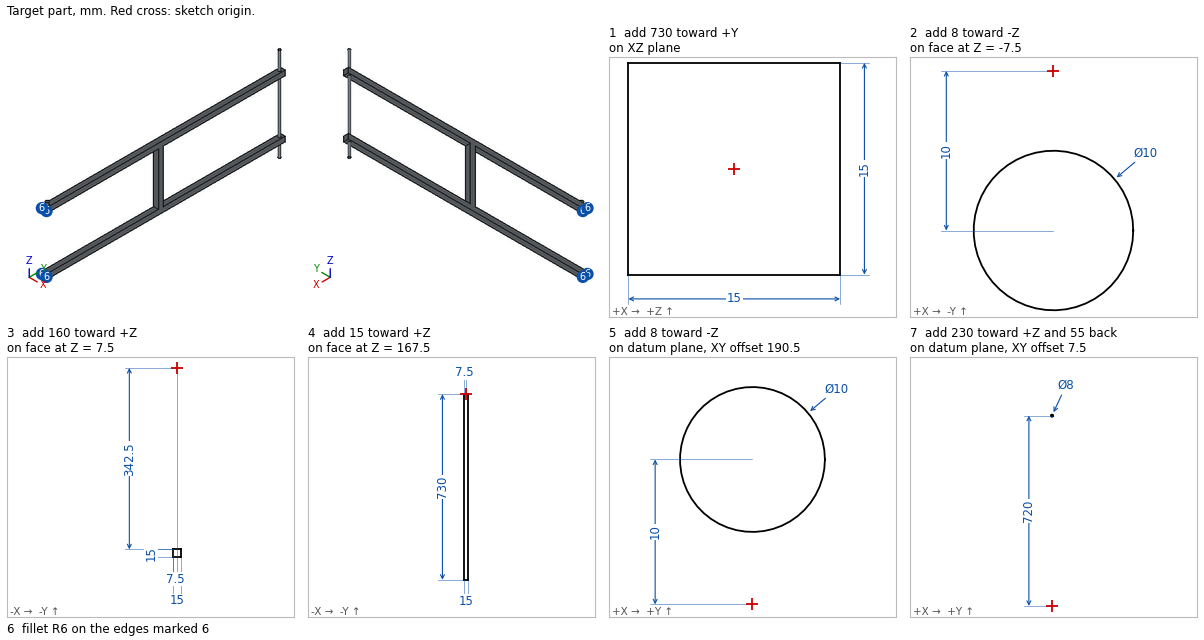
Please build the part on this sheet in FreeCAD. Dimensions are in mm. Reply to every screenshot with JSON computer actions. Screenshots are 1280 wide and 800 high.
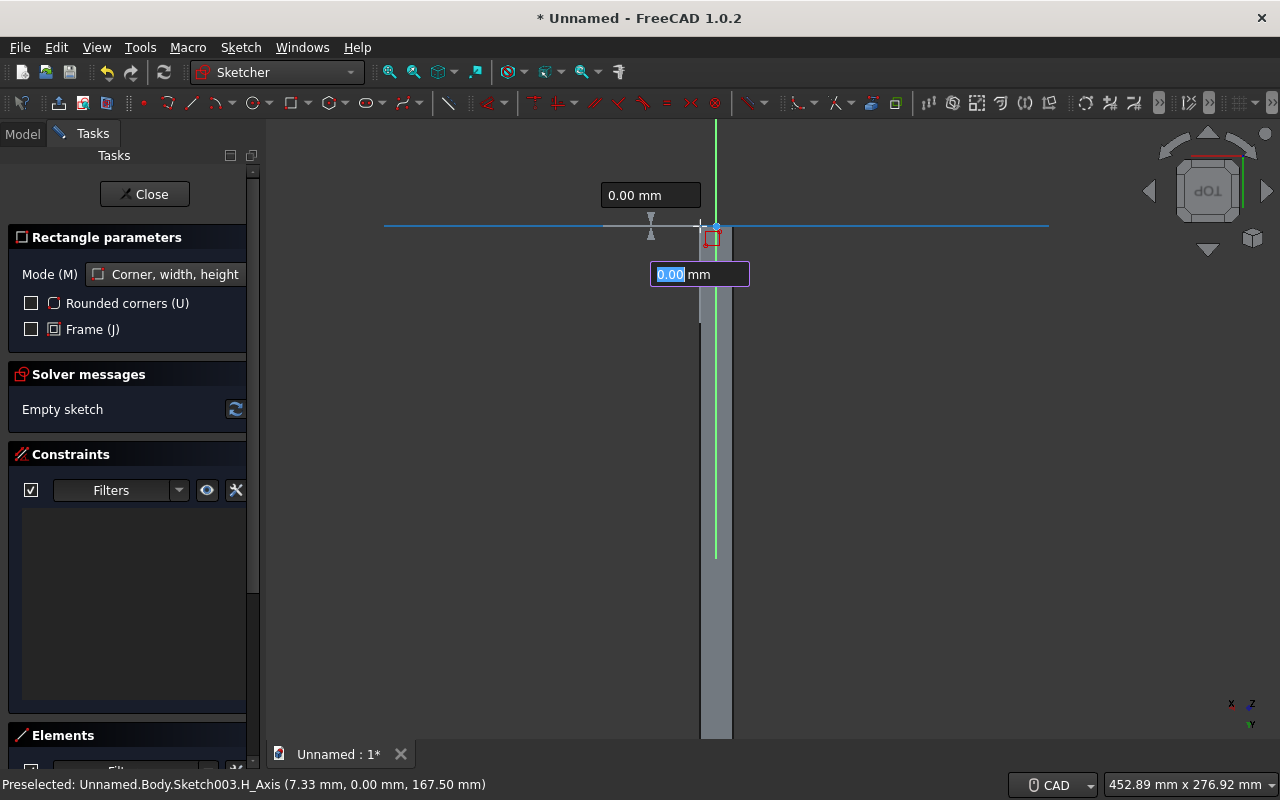
{"action": "scroll", "coordinate": [701, 228], "scroll_direction": "down", "scroll_amount": 7}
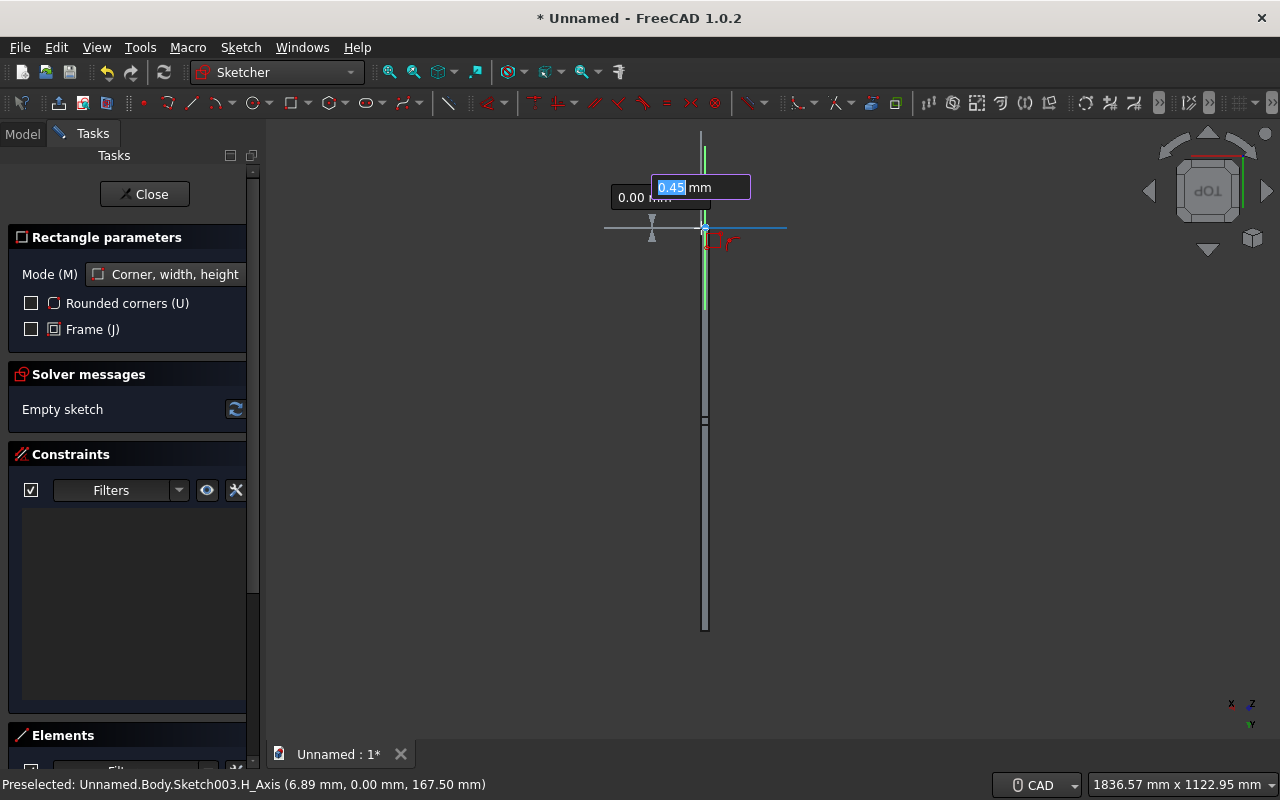
{"action": "scroll", "coordinate": [709, 631], "scroll_direction": "up", "scroll_amount": 7}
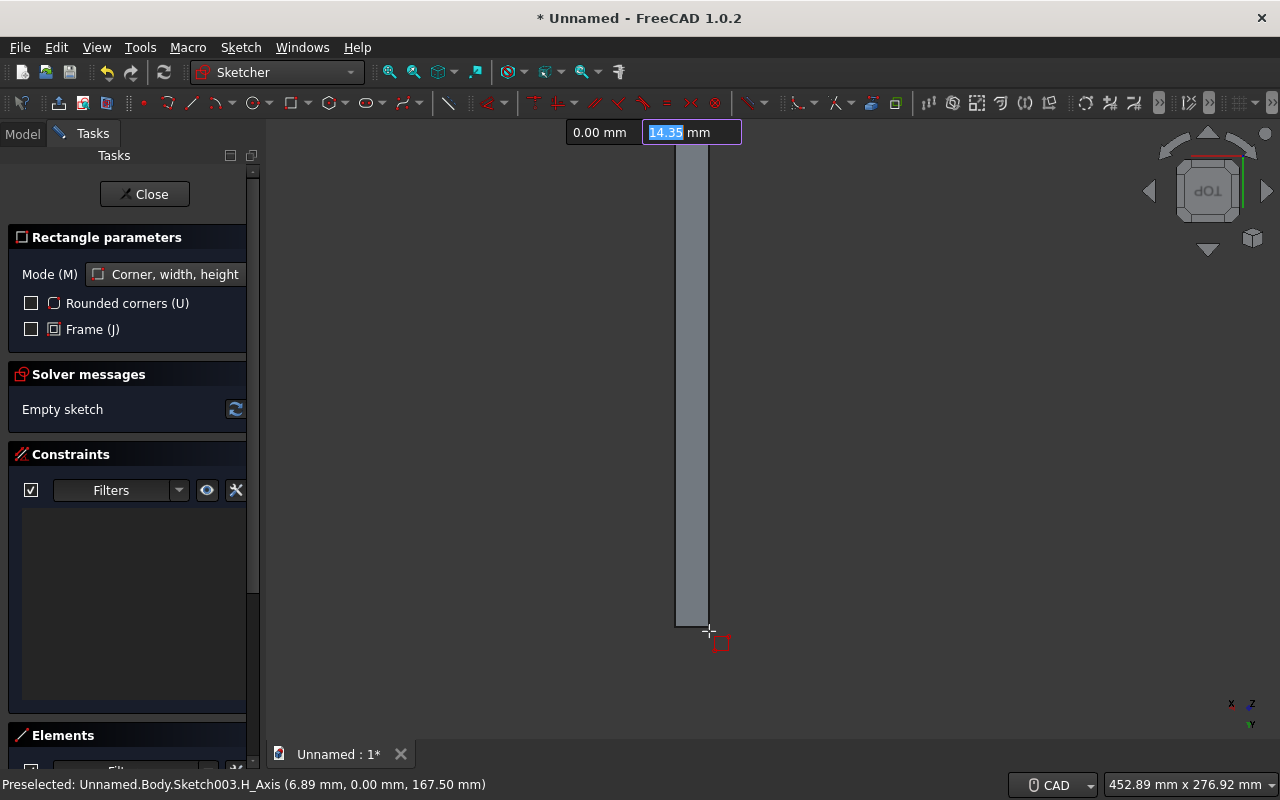
{"action": "left_click", "coordinate": [709, 627]}
{"action": "key", "text": "Escape"}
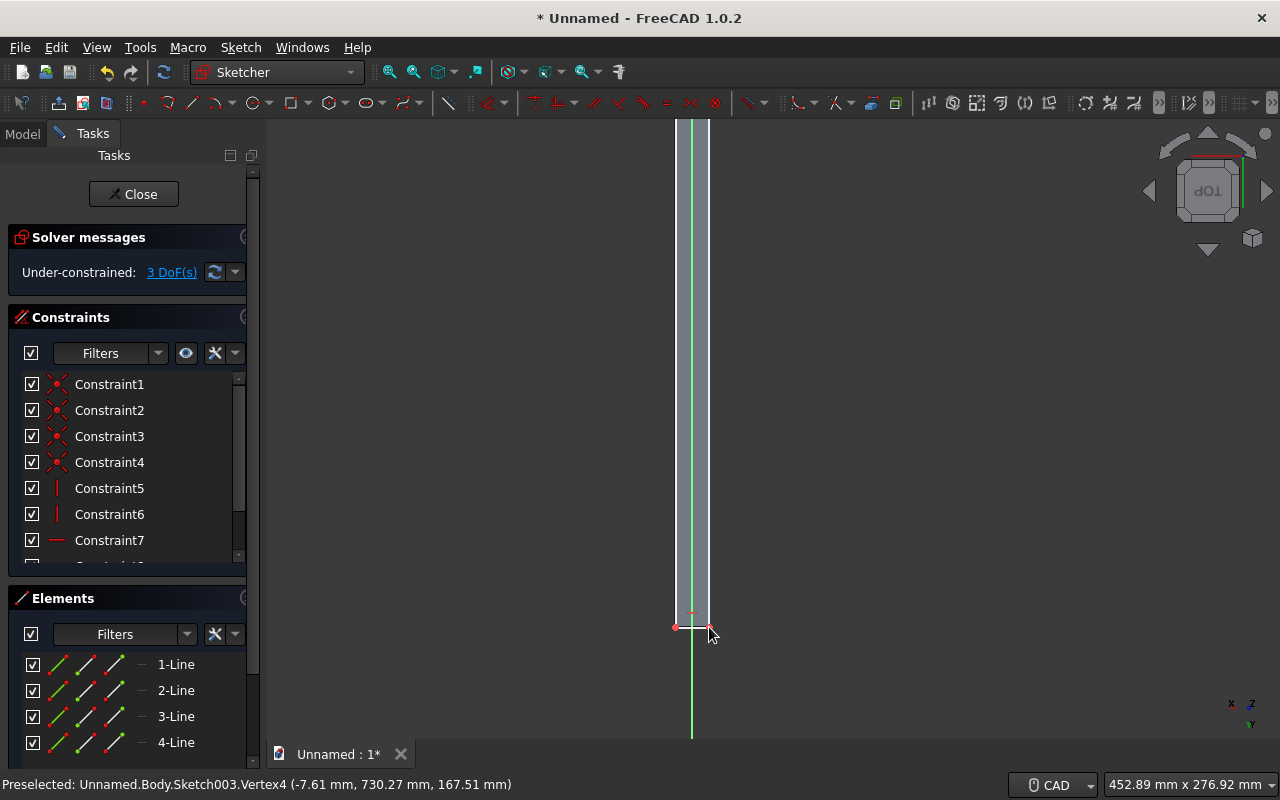
{"action": "left_click", "coordinate": [488, 104]}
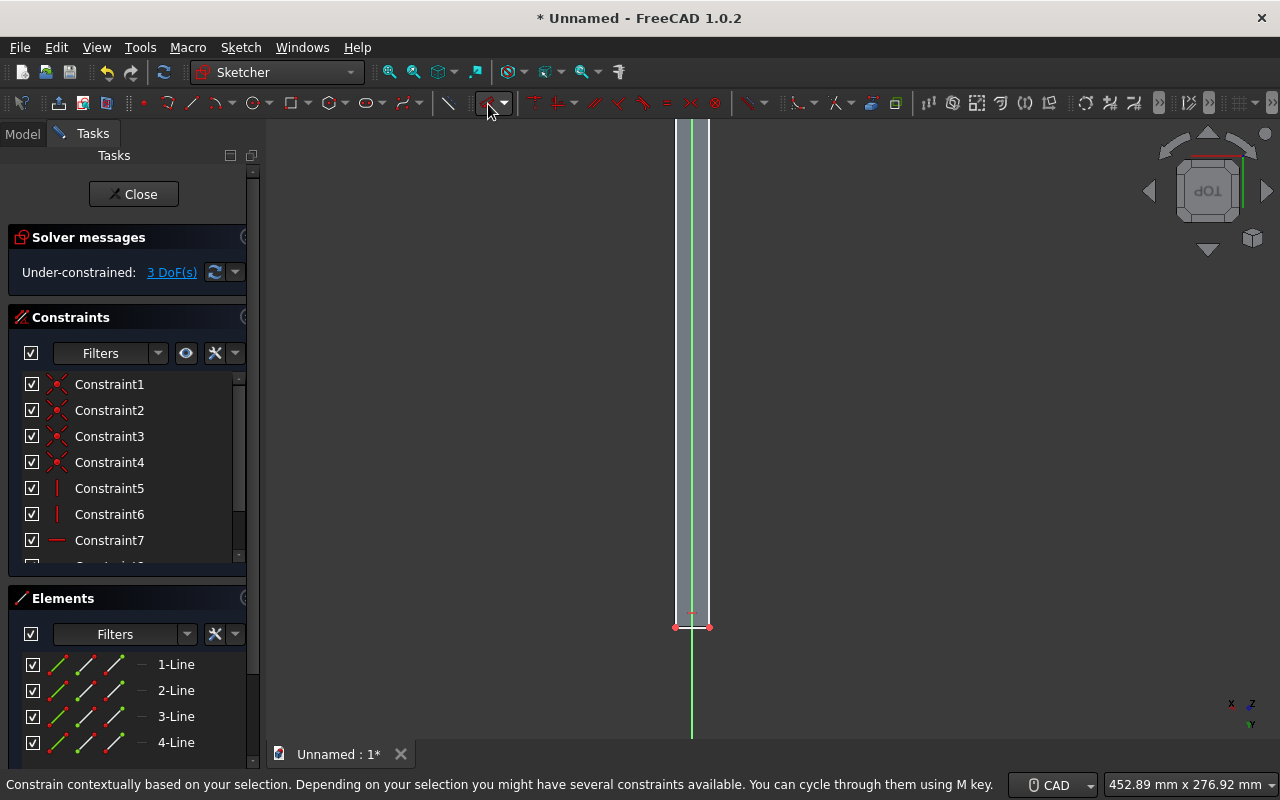
{"action": "left_click", "coordinate": [689, 628]}
{"action": "left_click", "coordinate": [685, 662]}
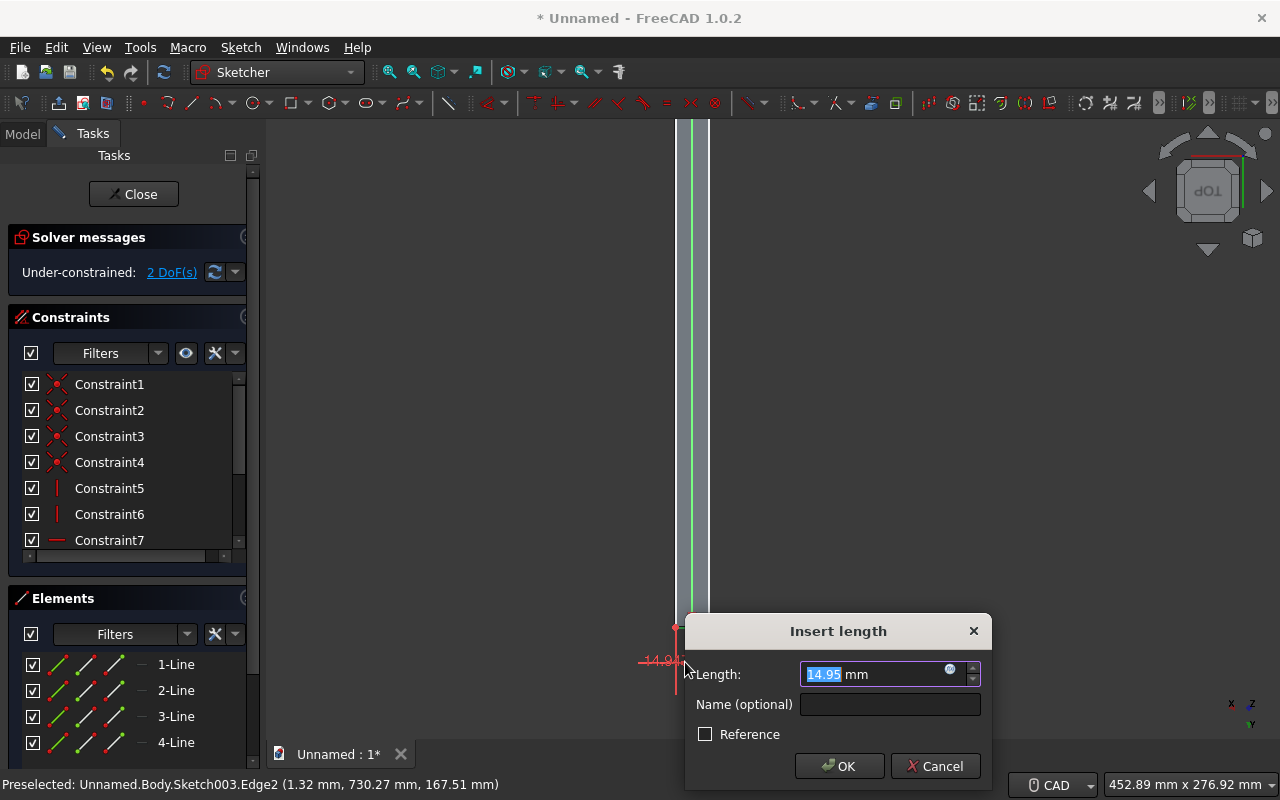
{"action": "type", "text": "15"}
{"action": "key", "text": "Return"}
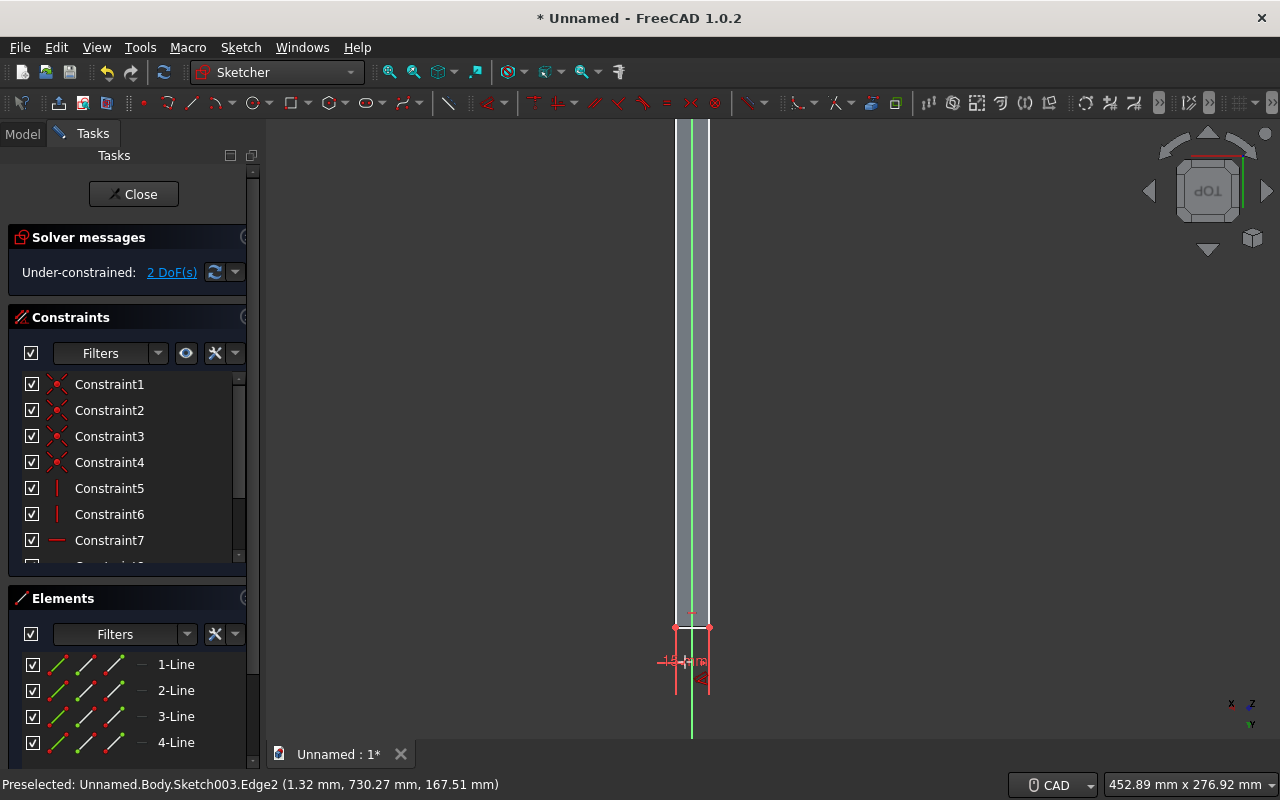
{"action": "left_click", "coordinate": [676, 301]}
{"action": "left_click", "coordinate": [642, 387]}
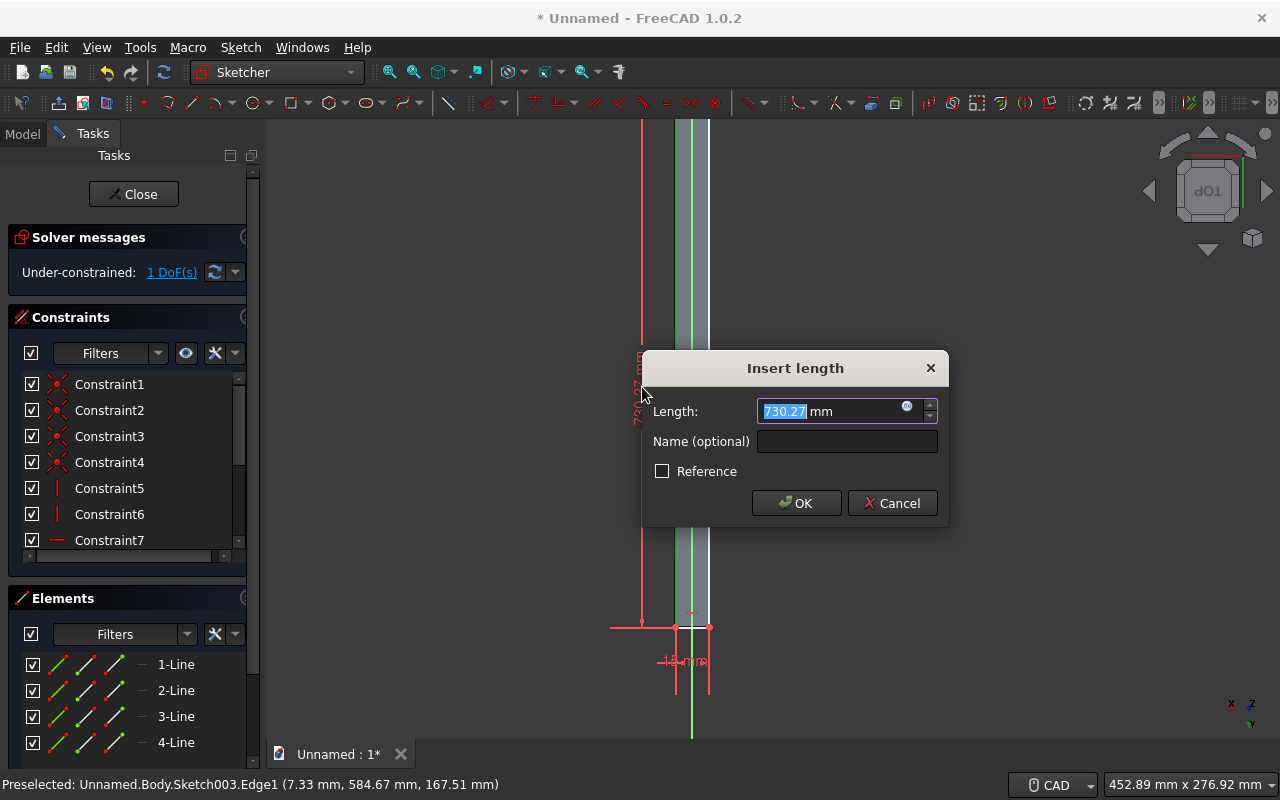
{"action": "type", "text": "730"}
{"action": "key", "text": "Return"}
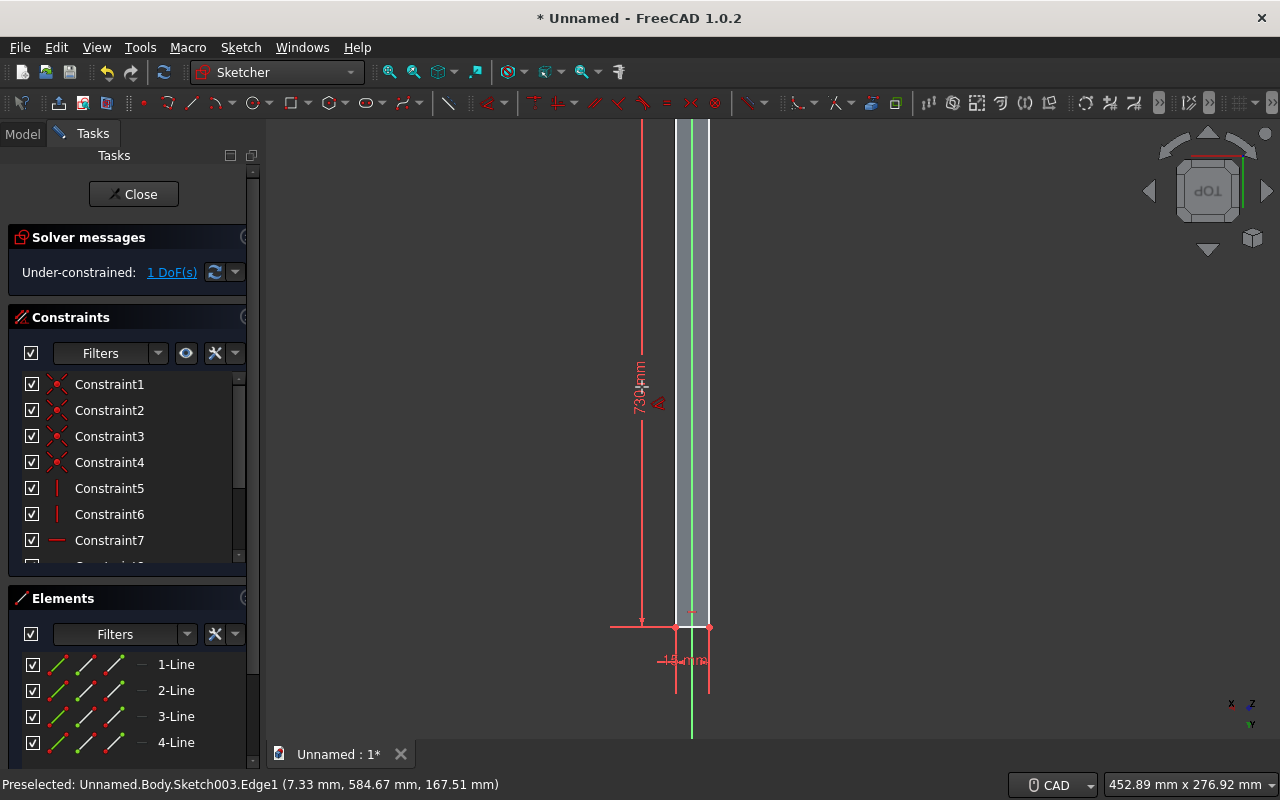
{"action": "scroll", "coordinate": [709, 632], "scroll_direction": "down", "scroll_amount": 7}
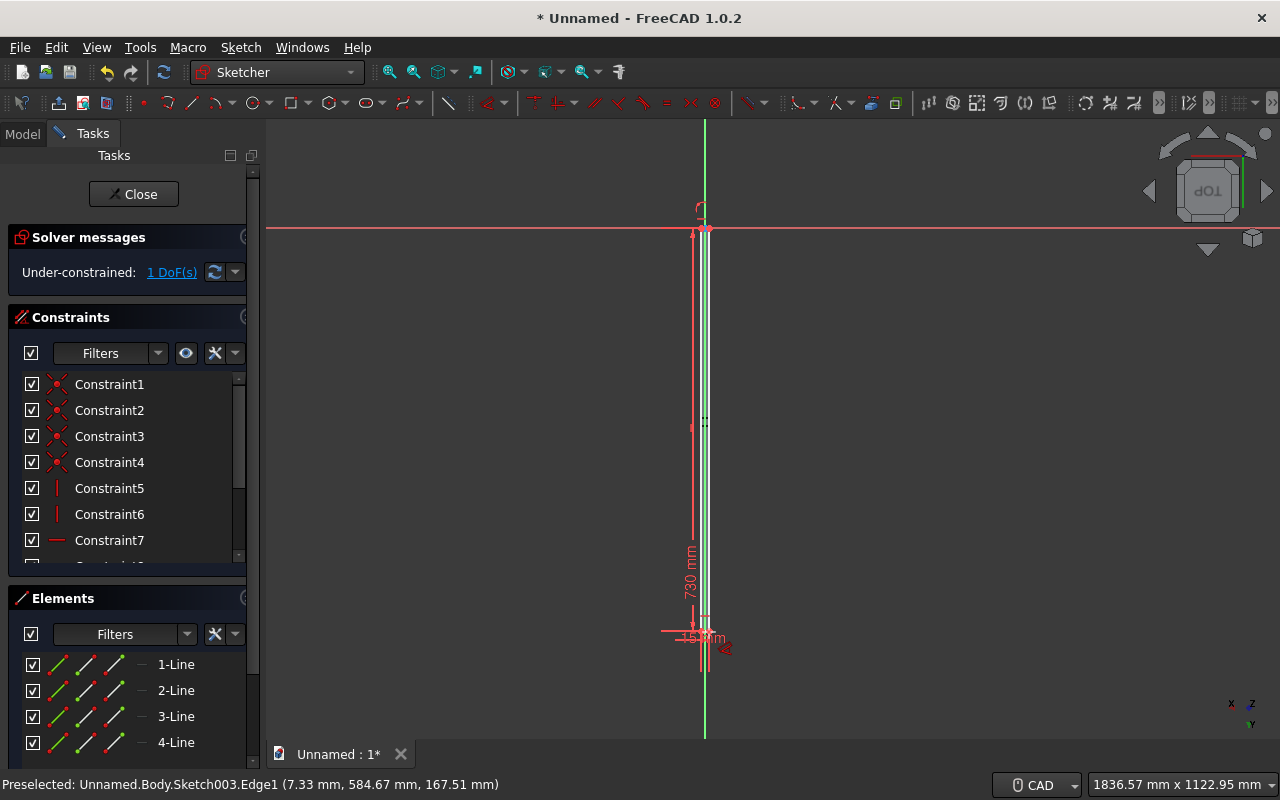
{"action": "scroll", "coordinate": [701, 228], "scroll_direction": "up", "scroll_amount": 12}